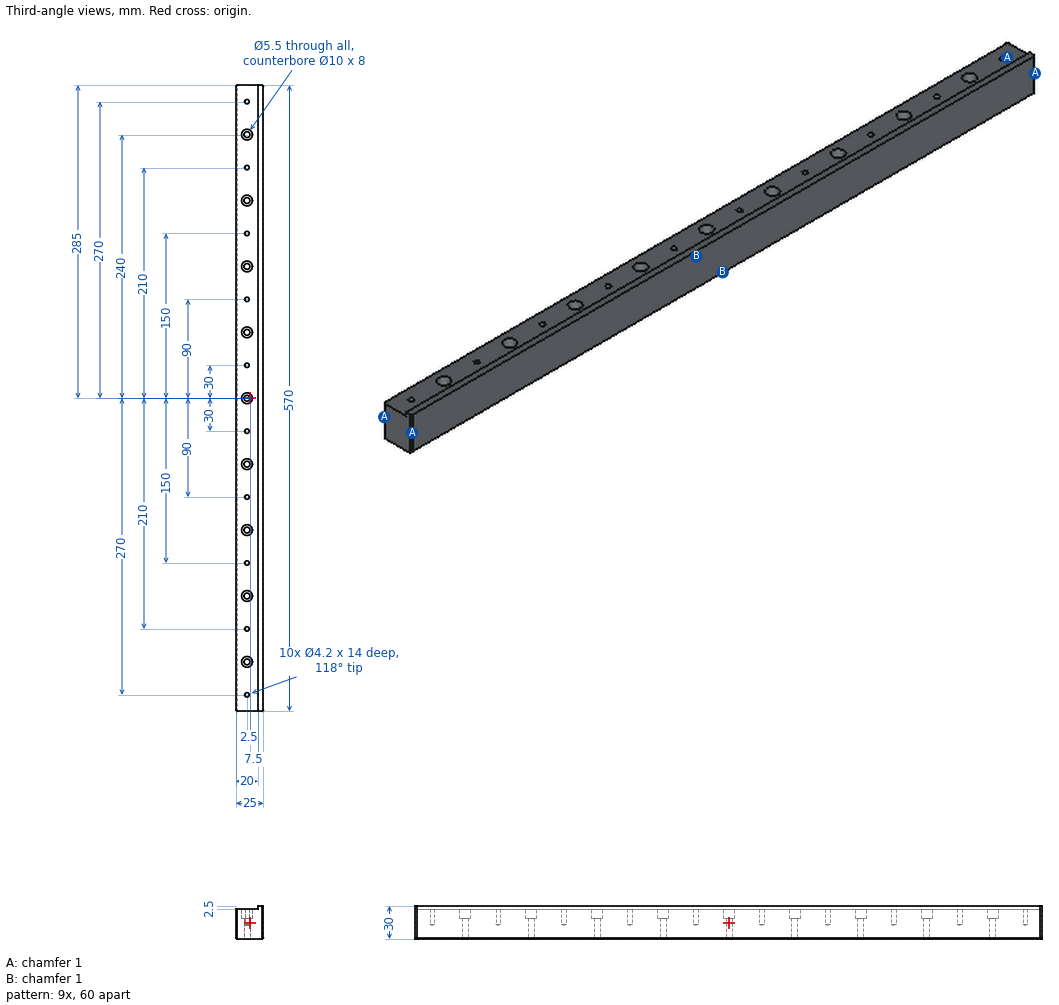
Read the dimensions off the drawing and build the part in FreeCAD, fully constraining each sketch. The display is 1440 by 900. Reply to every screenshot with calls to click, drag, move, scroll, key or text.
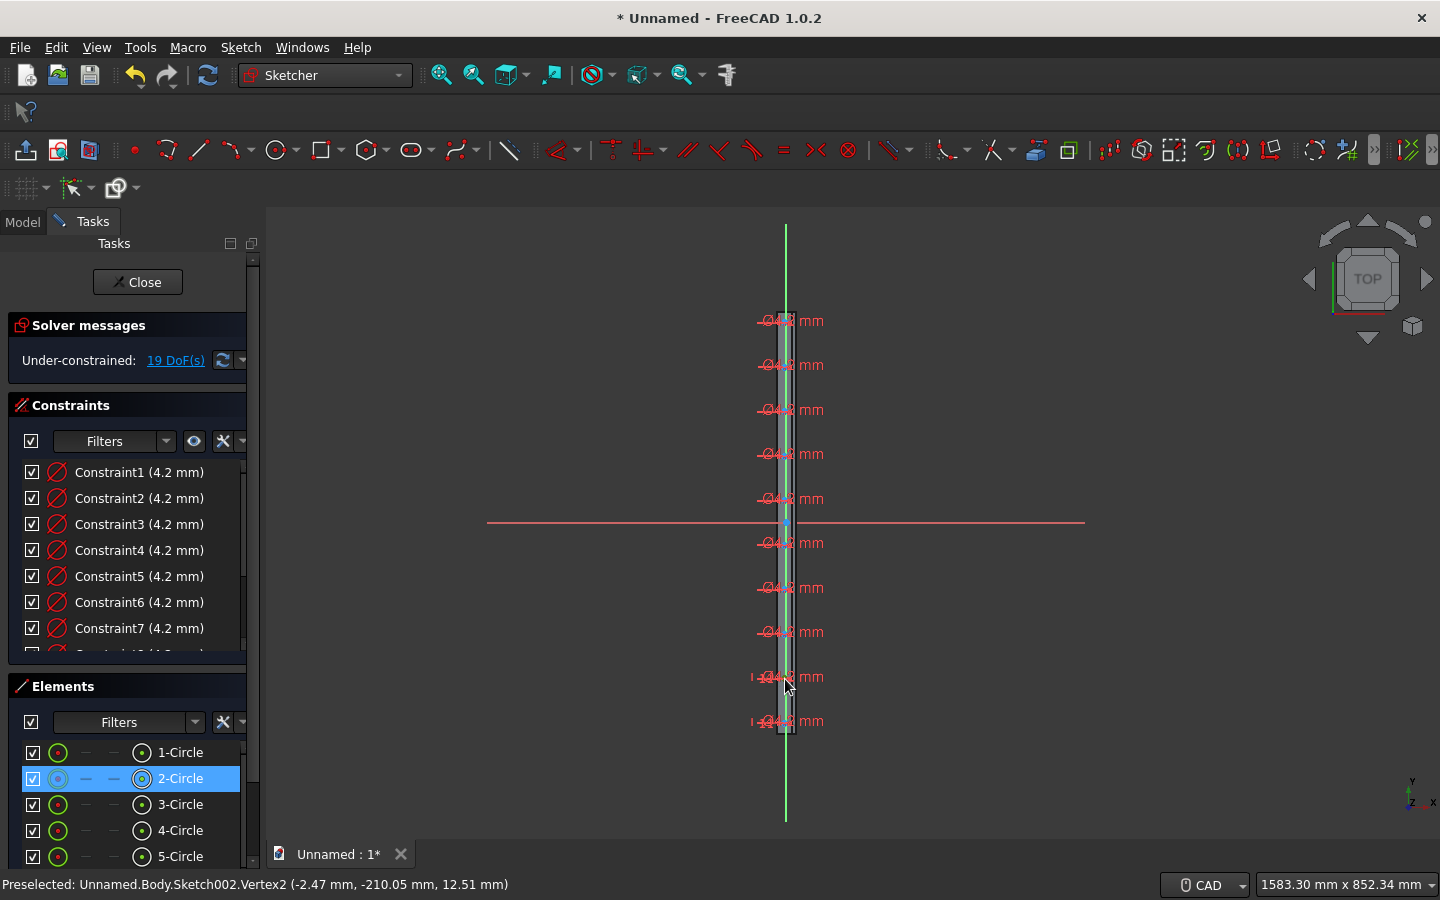
click(785, 634)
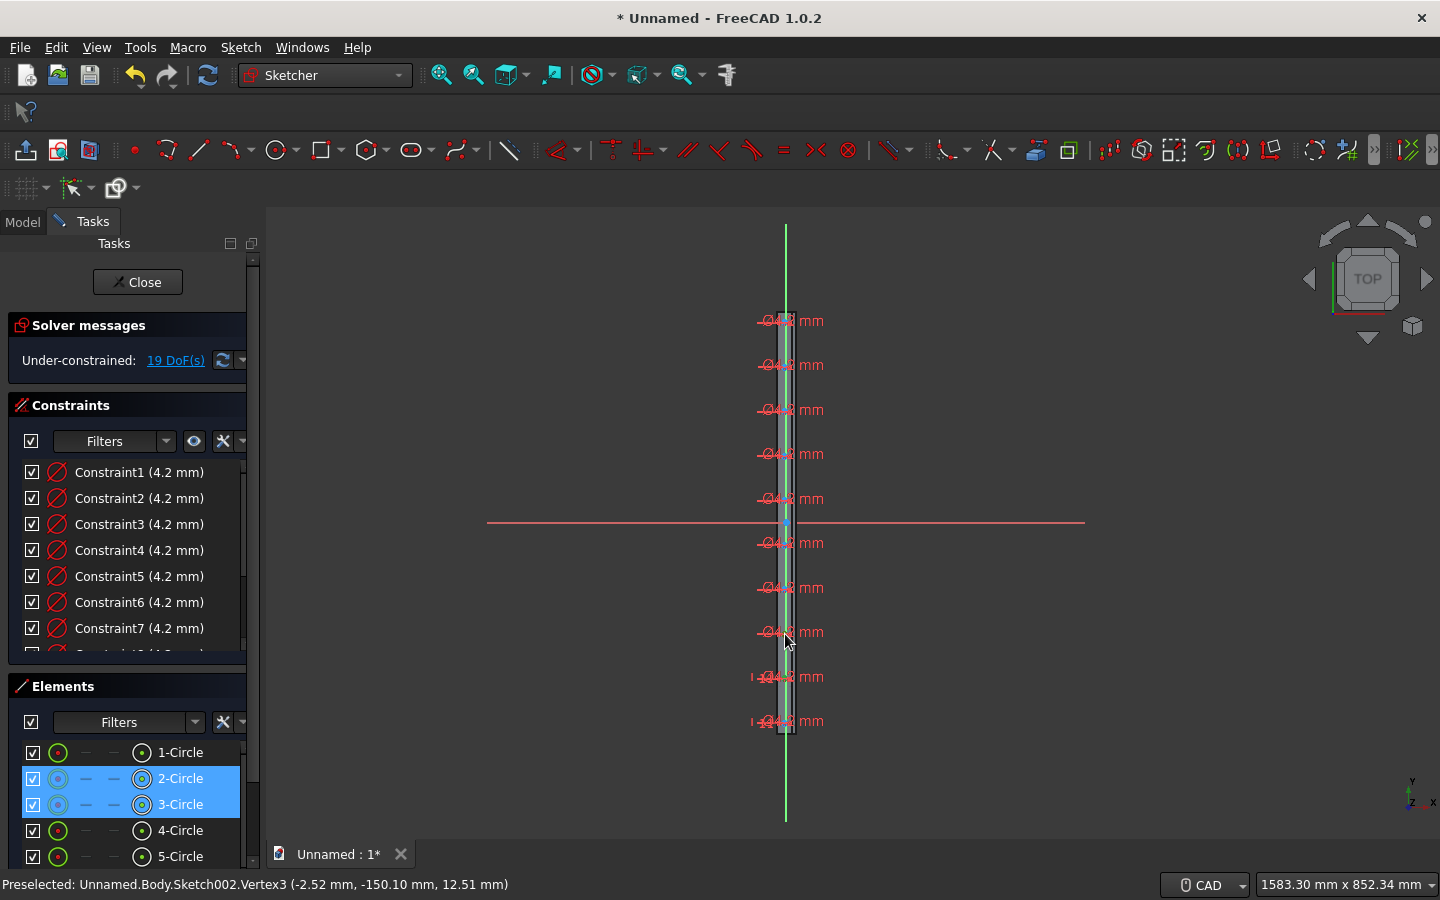
key(v)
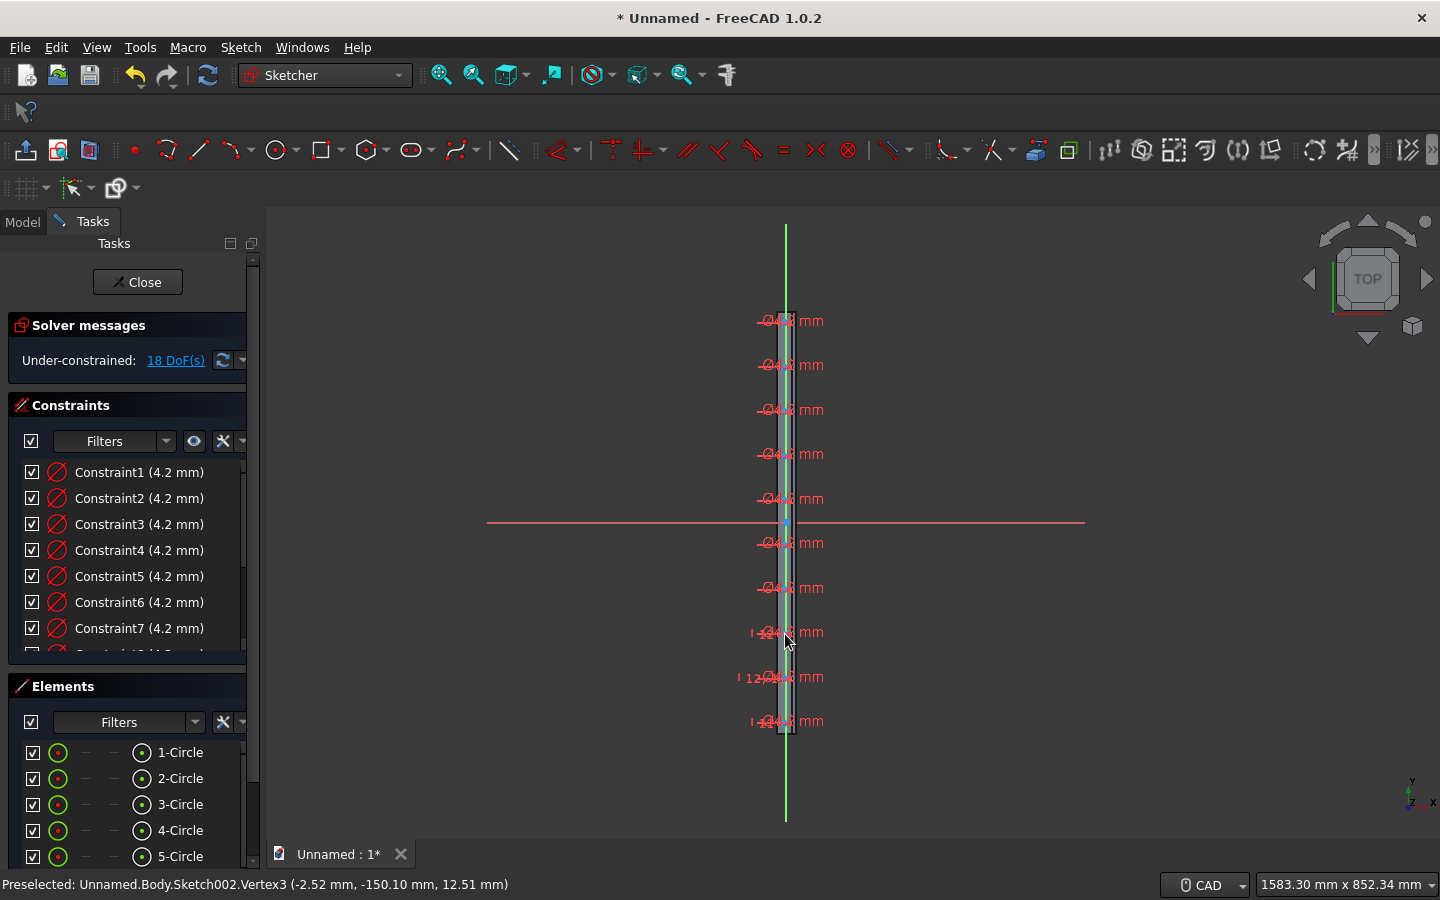
click(785, 634)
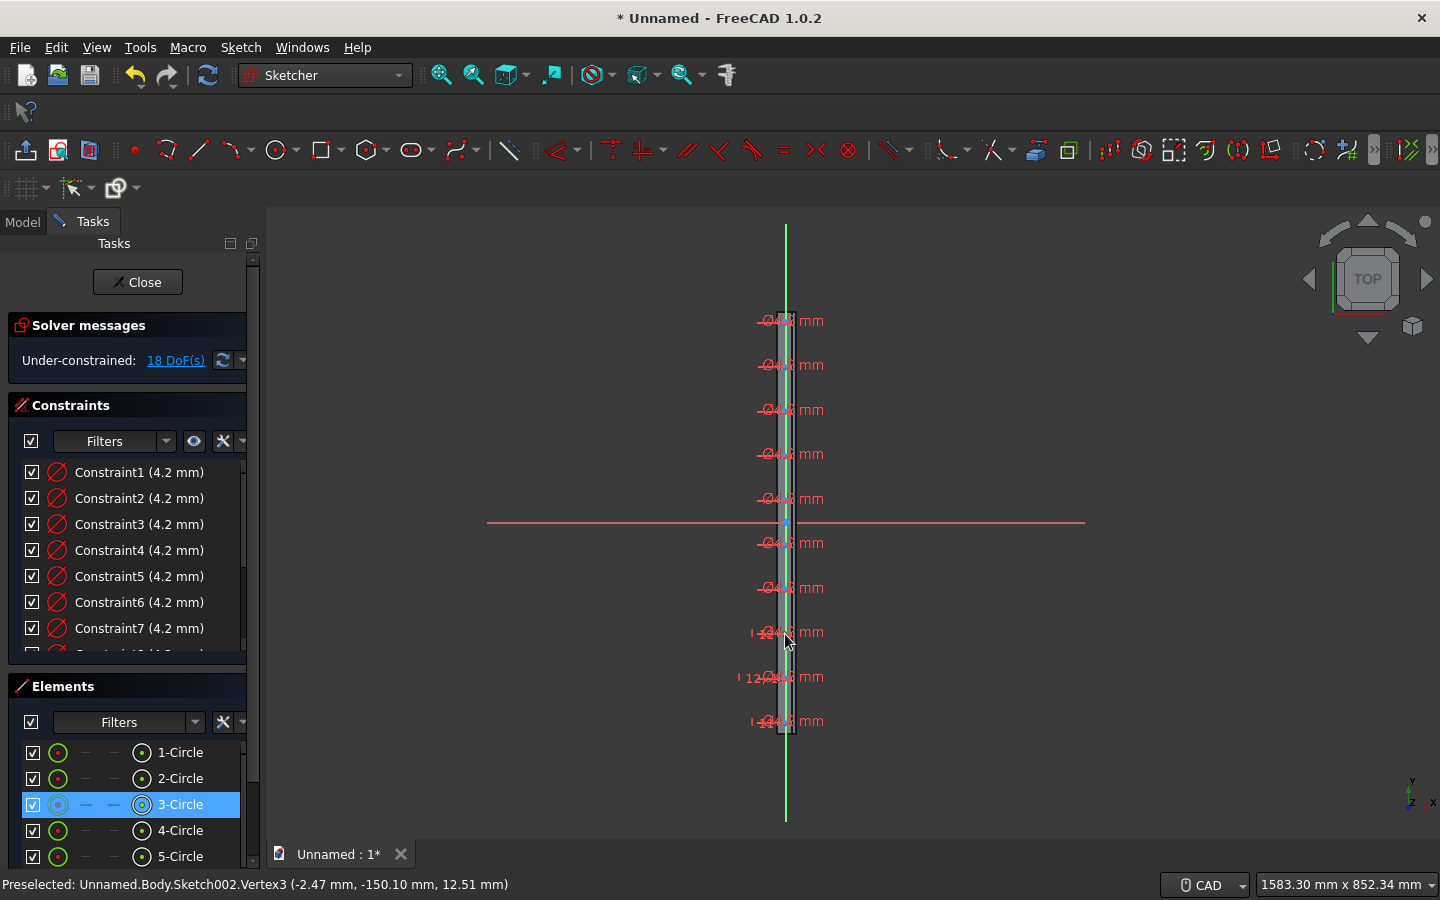
click(785, 590)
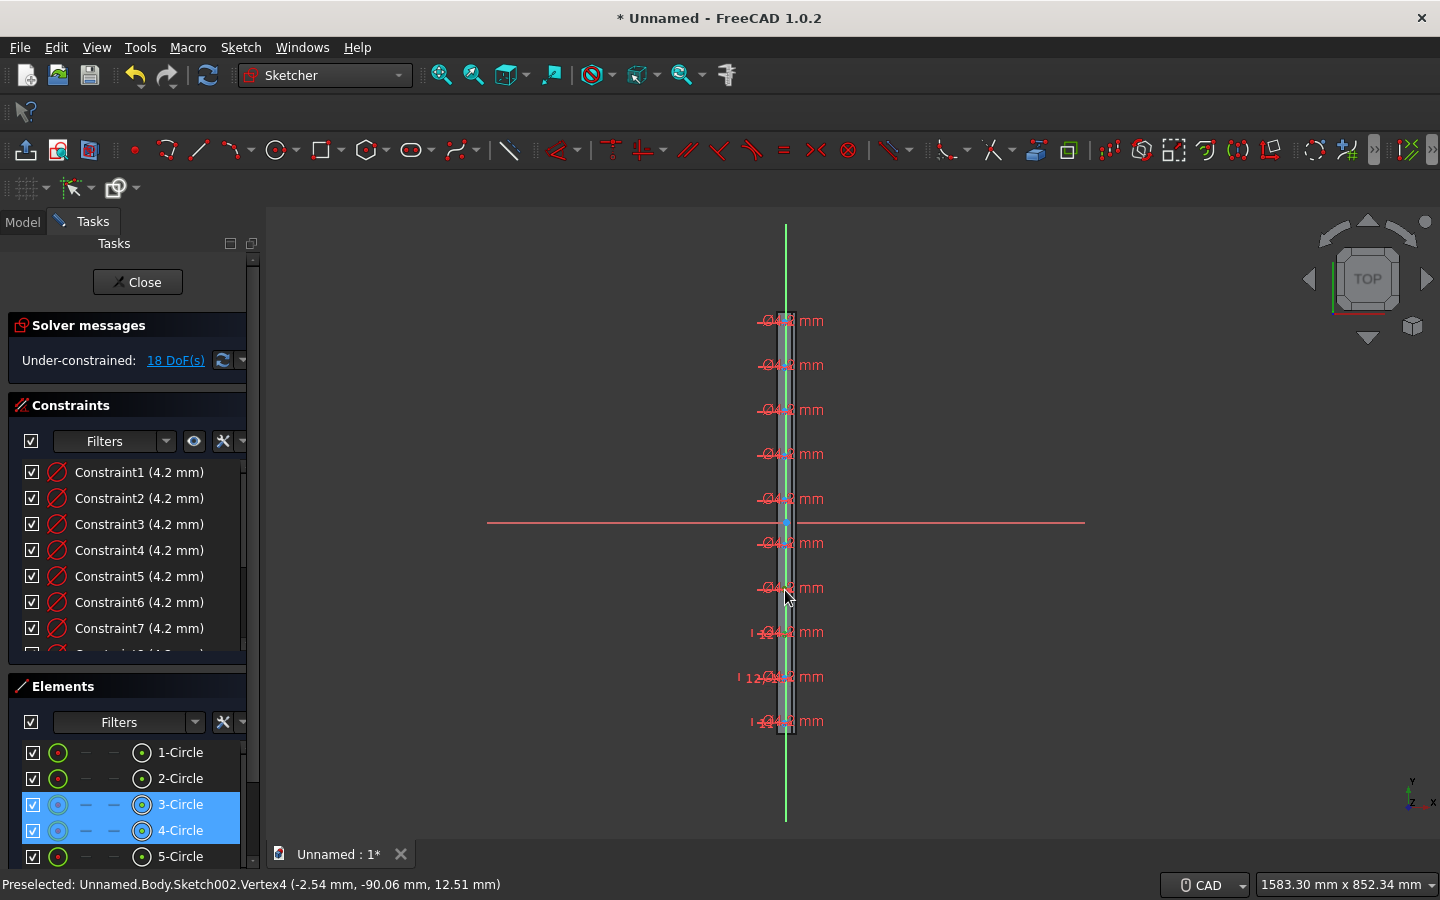
key(v)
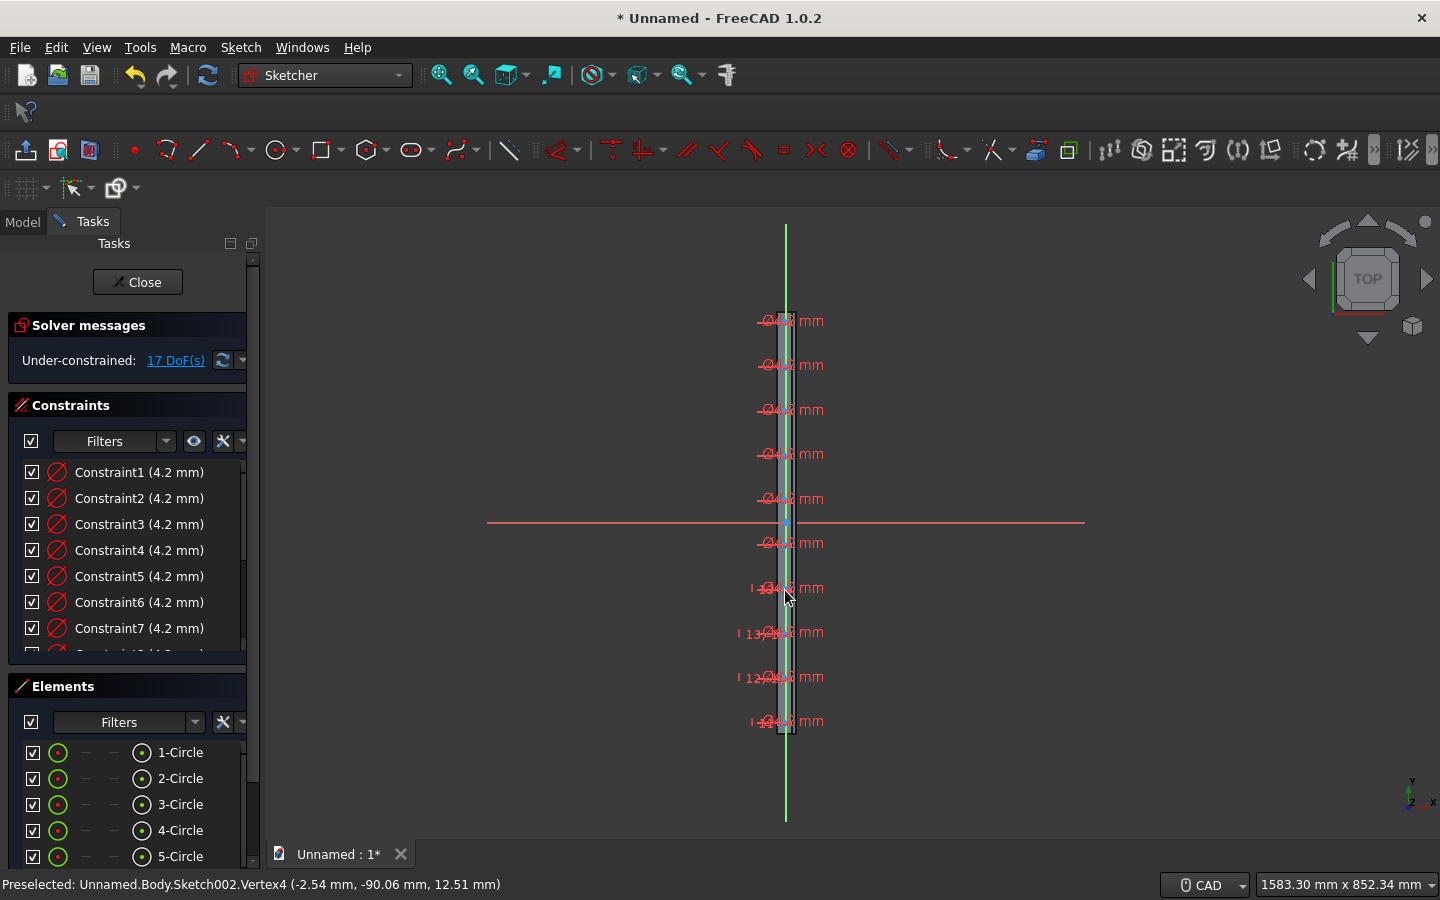
click(785, 590)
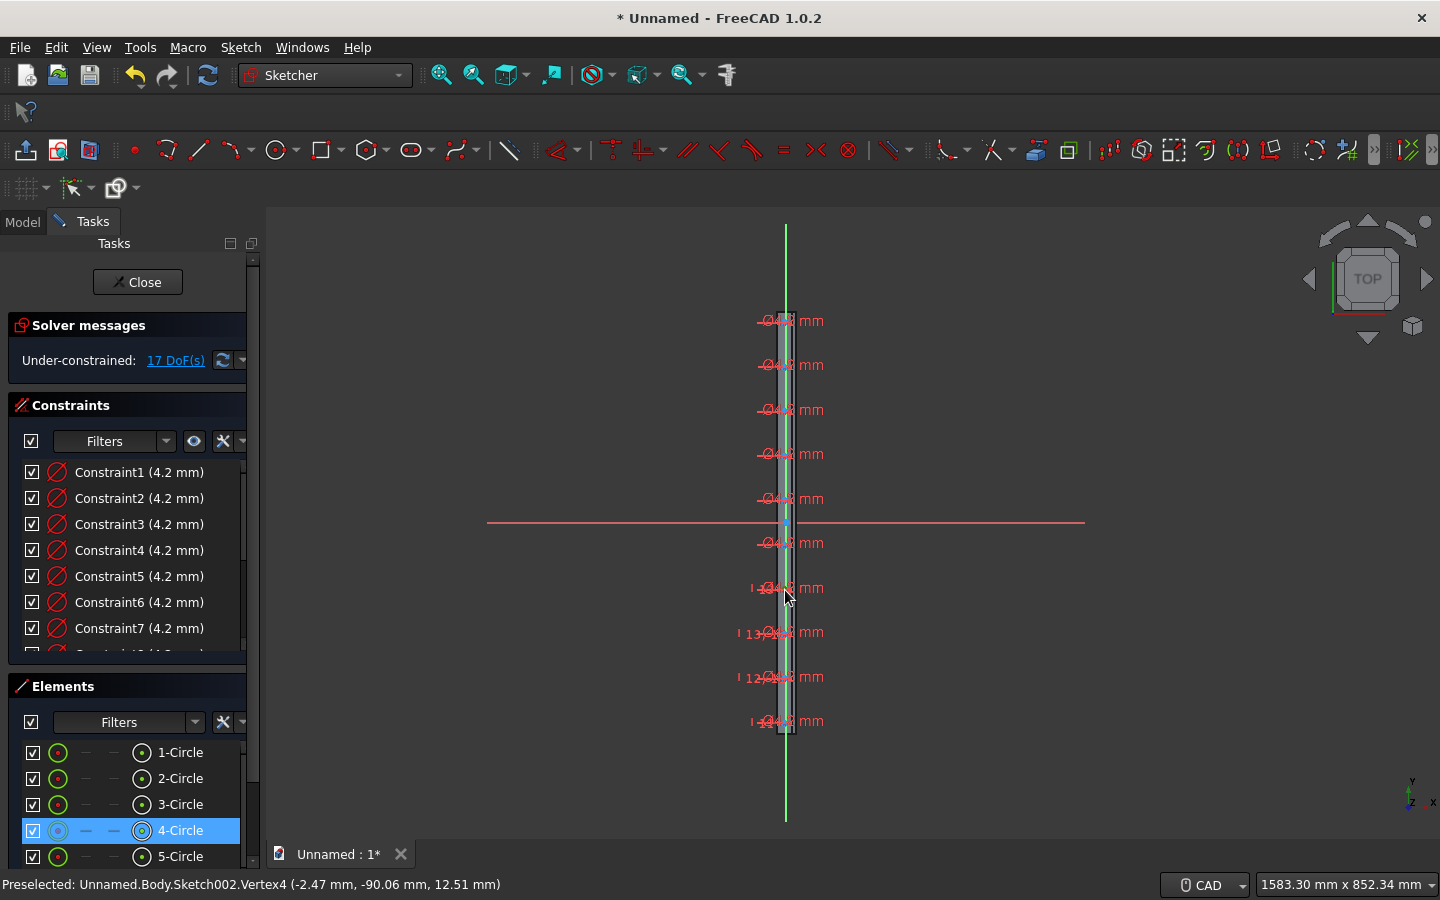
click(785, 545)